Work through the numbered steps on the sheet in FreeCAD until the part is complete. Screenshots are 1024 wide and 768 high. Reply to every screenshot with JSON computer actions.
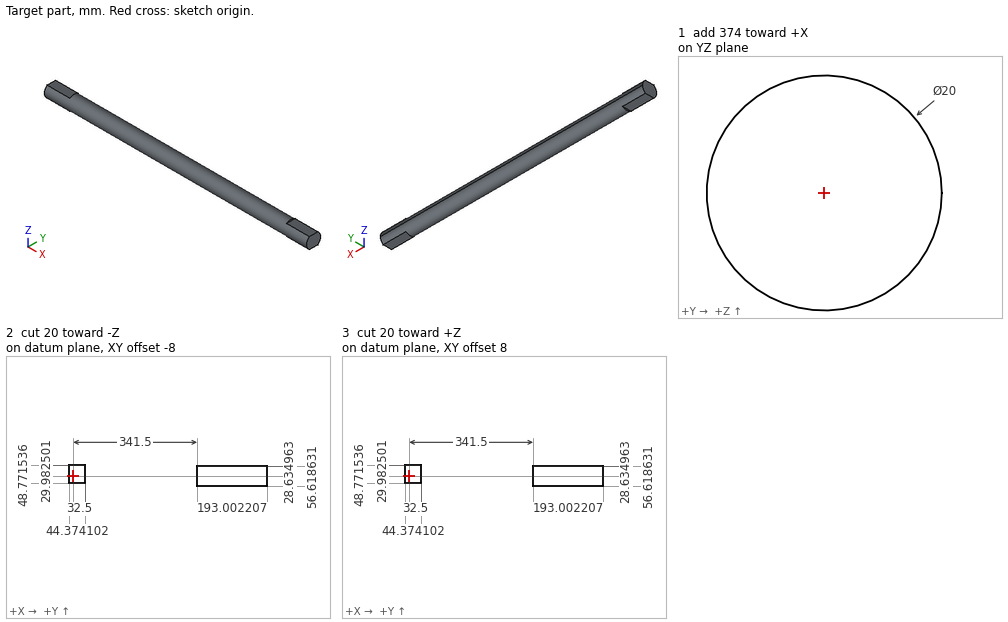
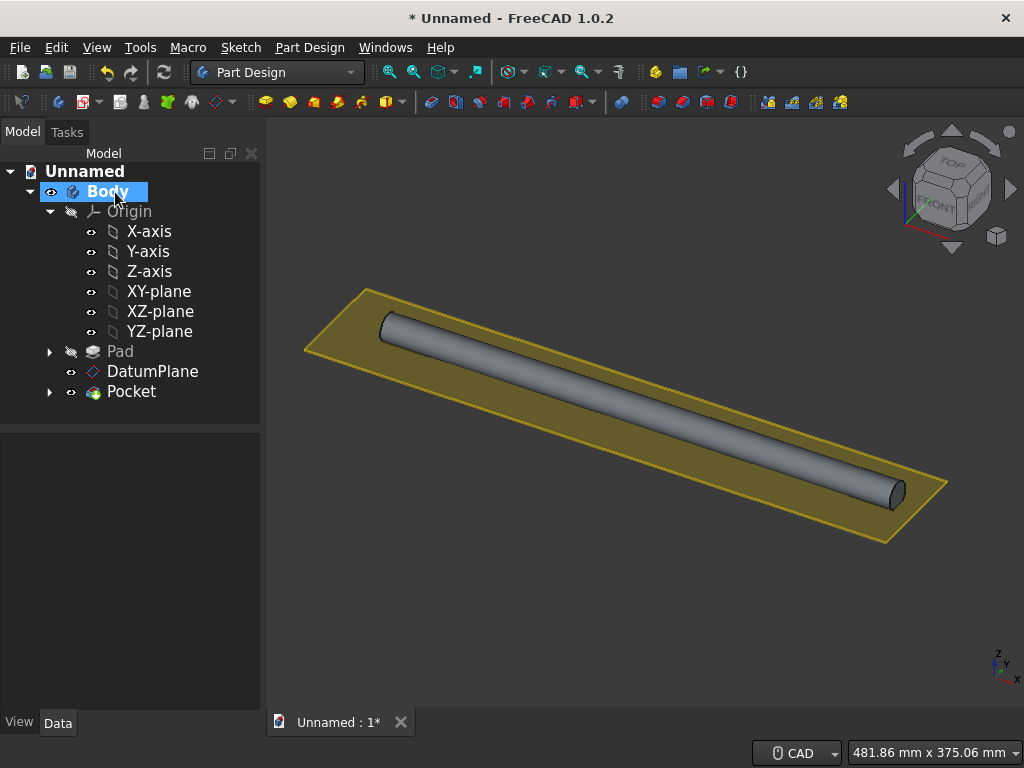
{"action": "left_click", "coordinate": [116, 372]}
{"action": "key", "text": "space"}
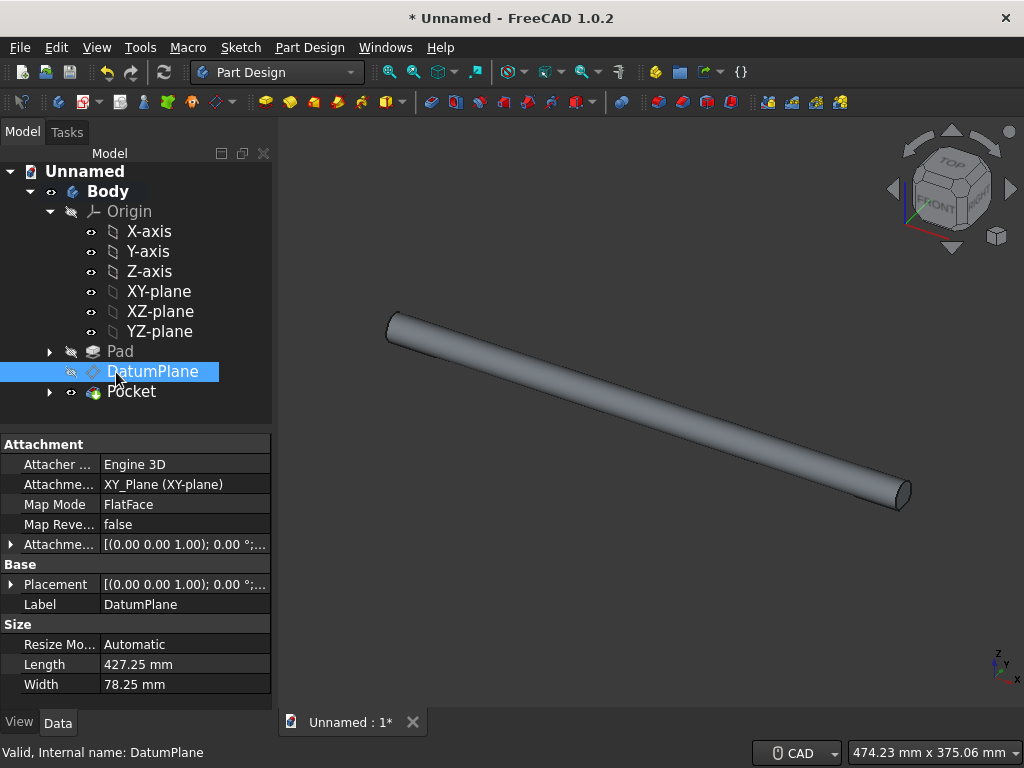
{"action": "left_click", "coordinate": [136, 292]}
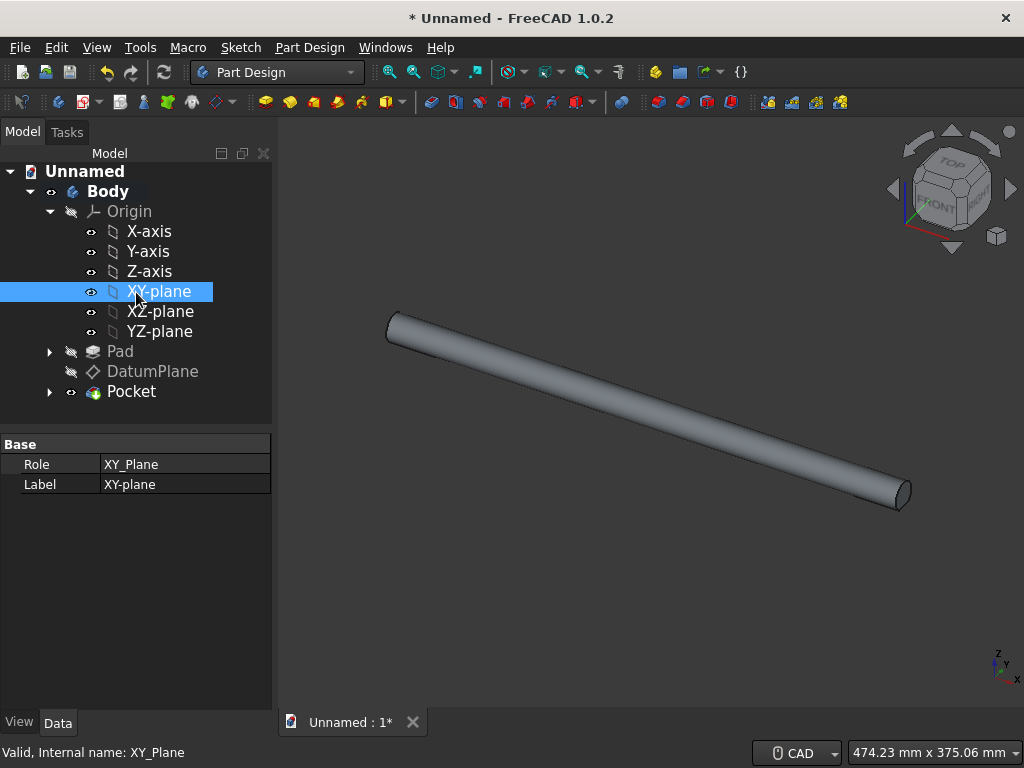
{"action": "left_click", "coordinate": [216, 102]}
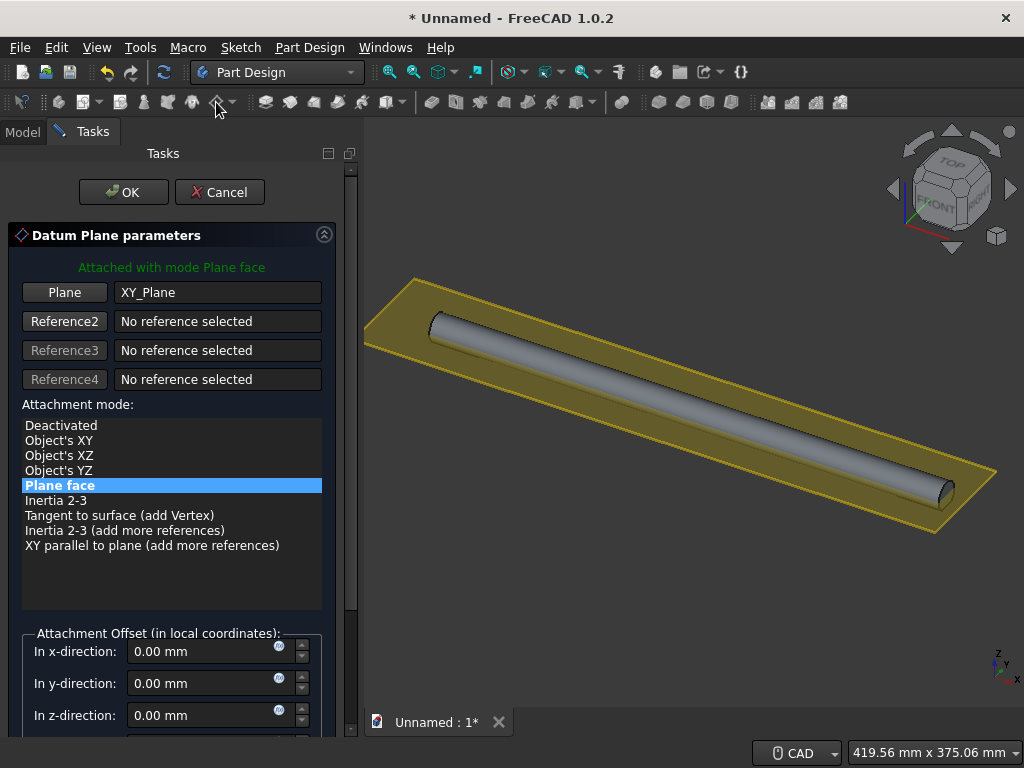
{"action": "triple_click", "coordinate": [210, 715]}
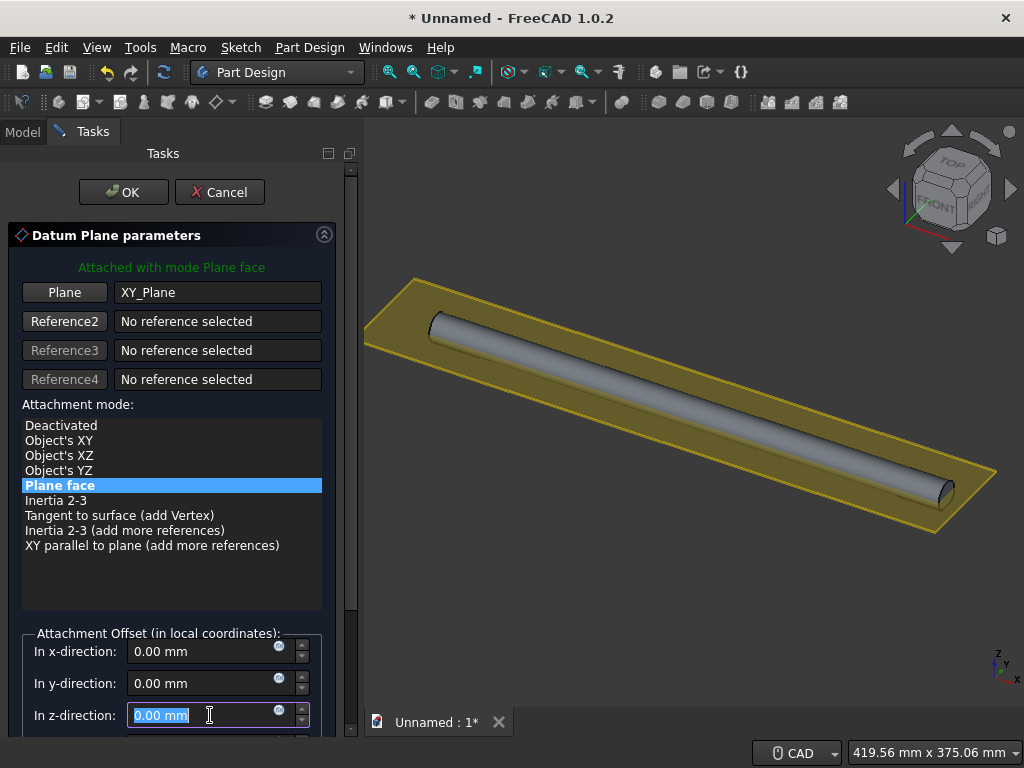
{"action": "type", "text": "8"}
{"action": "key", "text": "Tab"}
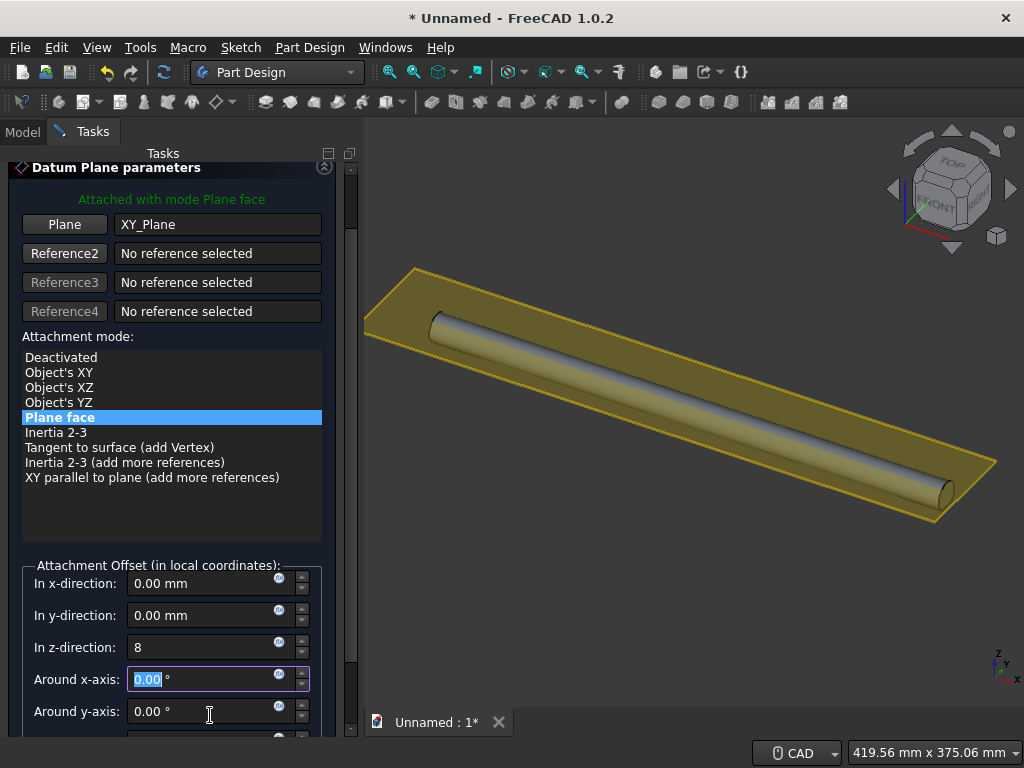
{"action": "scroll", "coordinate": [351, 450], "scroll_direction": "up", "scroll_amount": 2}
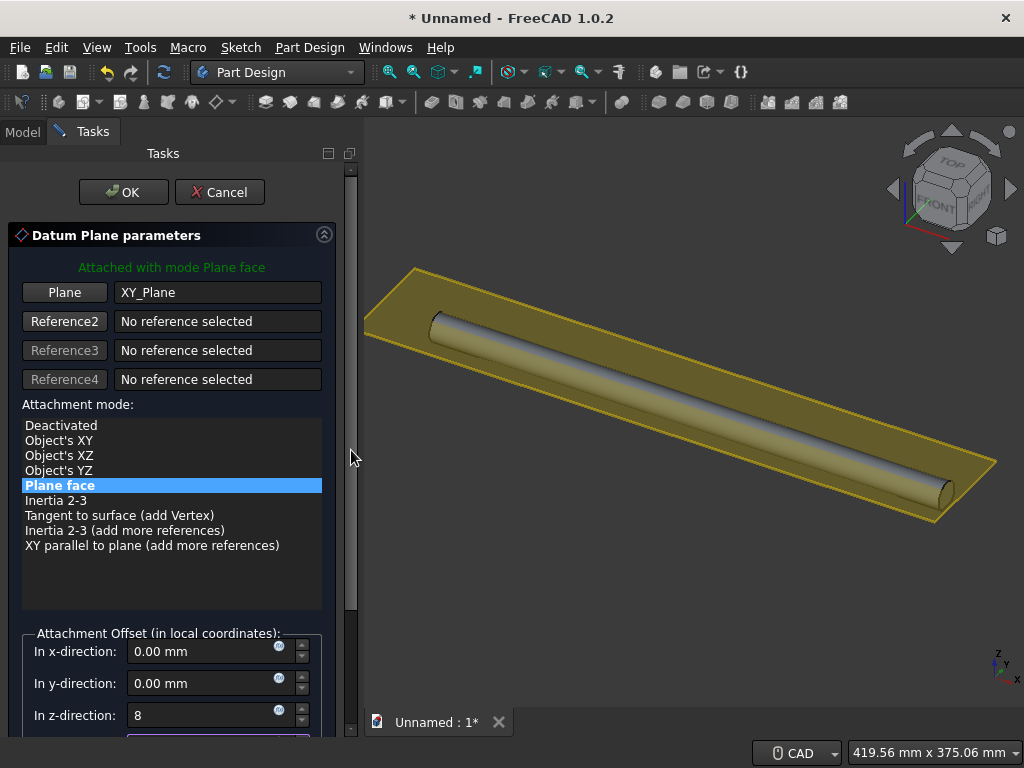
{"action": "left_click", "coordinate": [124, 192]}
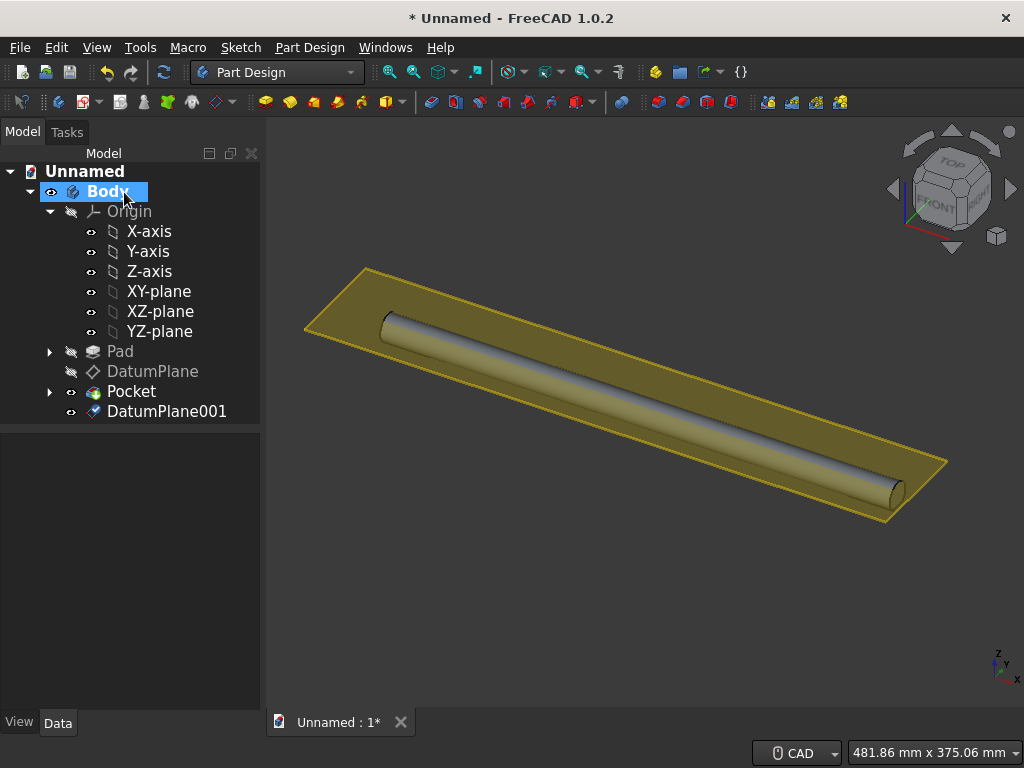
{"action": "left_click", "coordinate": [116, 412]}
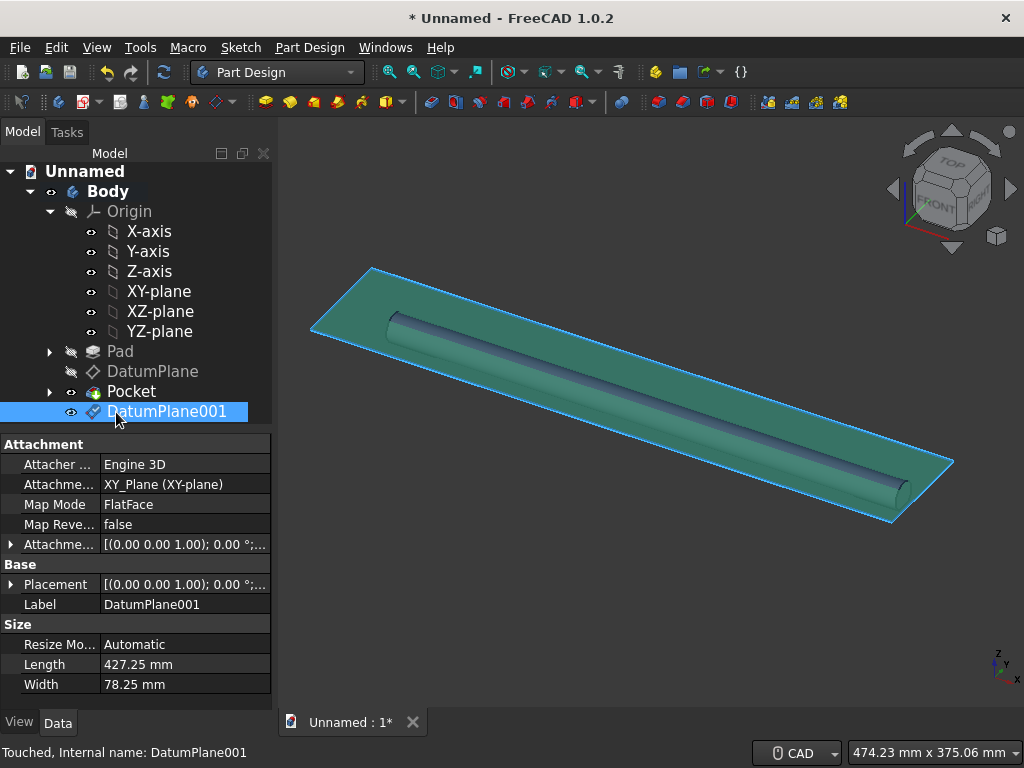
{"action": "left_click", "coordinate": [84, 102]}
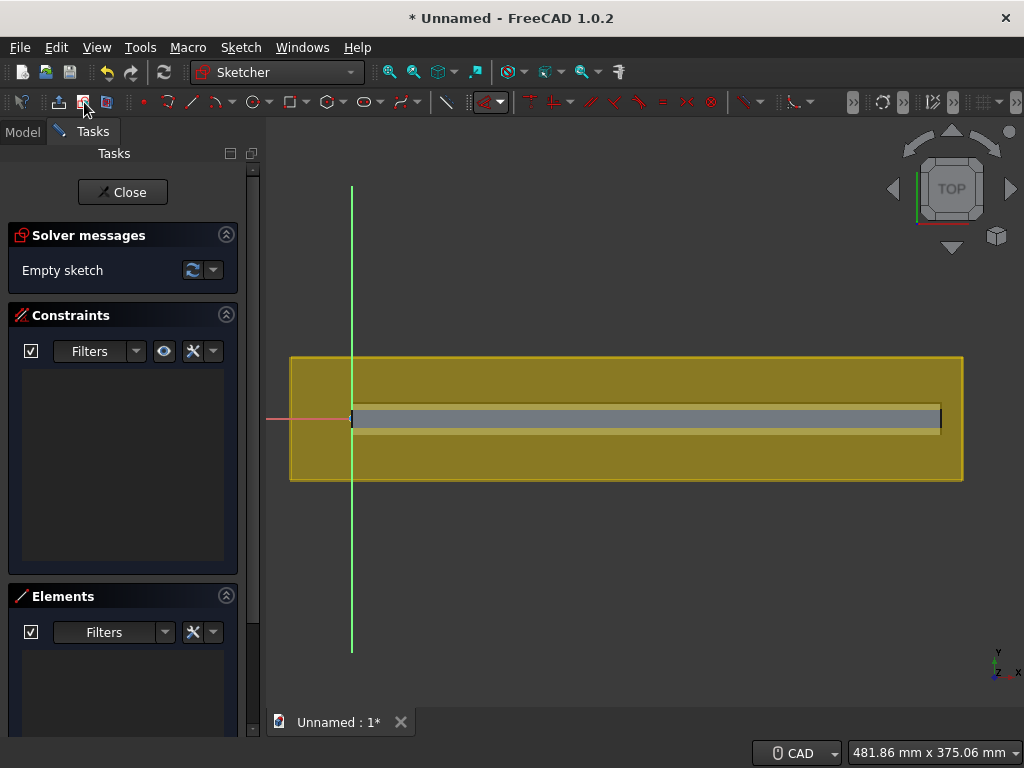
{"action": "key", "text": "q s"}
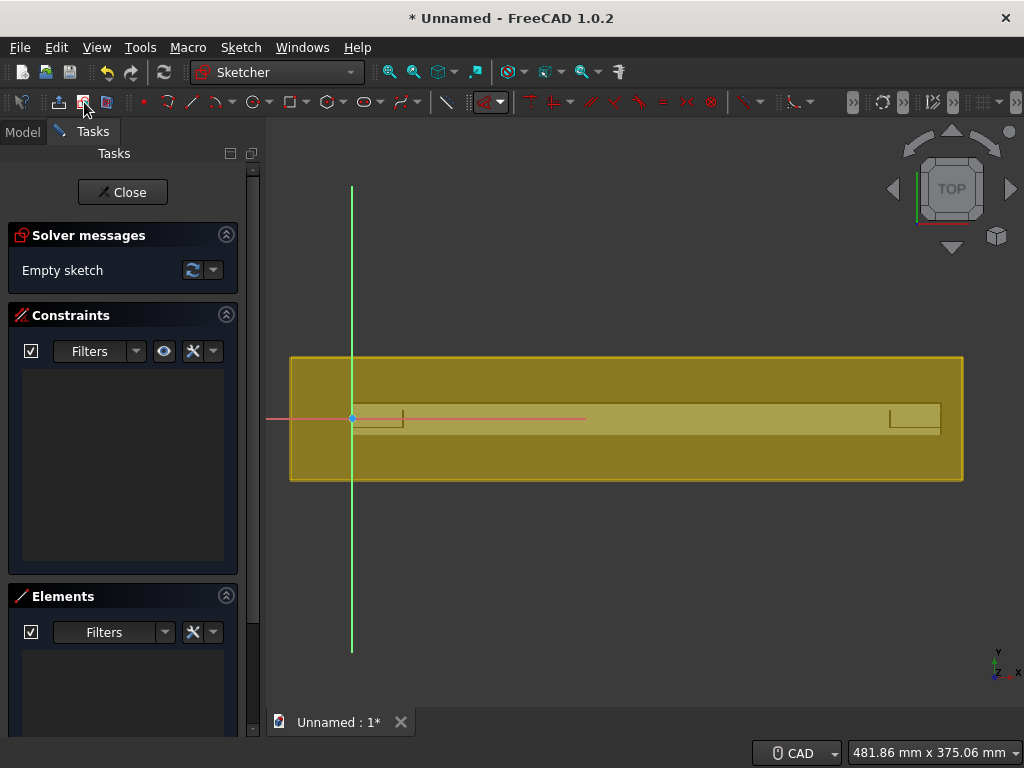
{"action": "scroll", "coordinate": [424, 408], "scroll_direction": "down", "scroll_amount": 4}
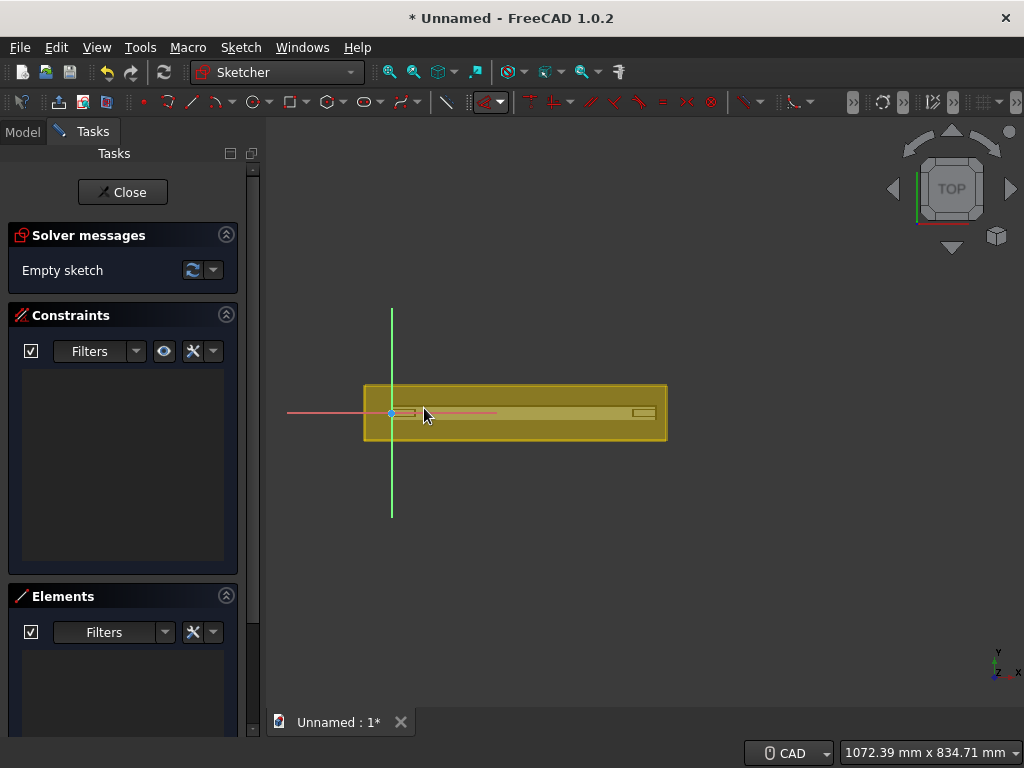
{"action": "left_click", "coordinate": [290, 102]}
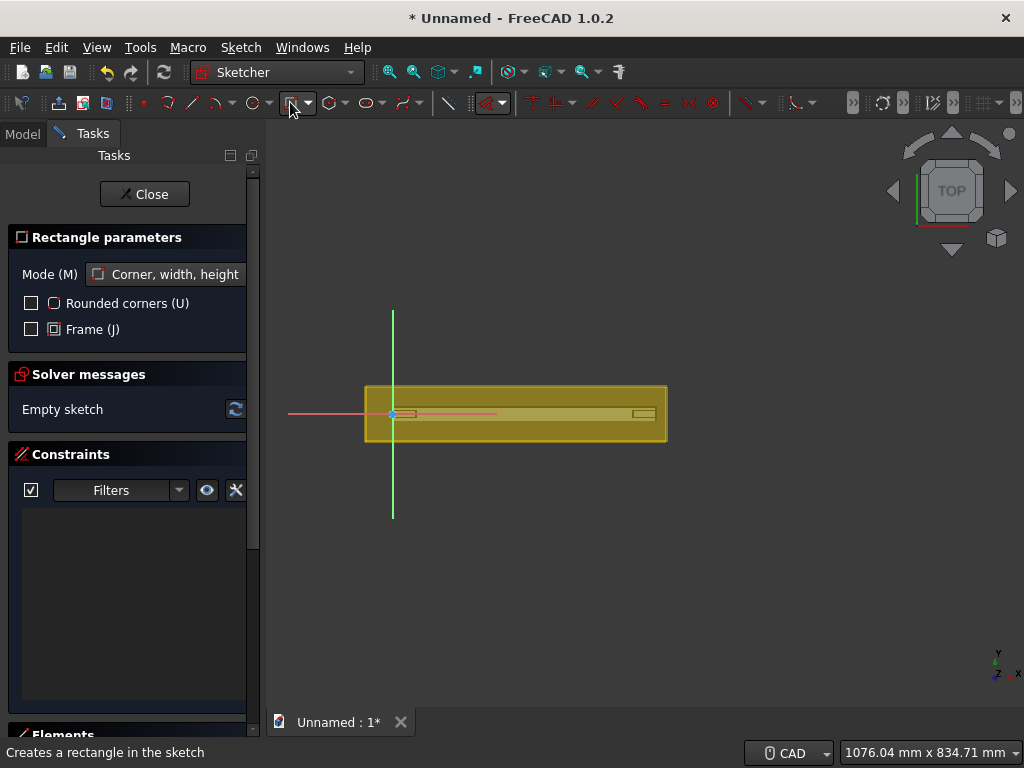
{"action": "scroll", "coordinate": [384, 393], "scroll_direction": "up", "scroll_amount": 4}